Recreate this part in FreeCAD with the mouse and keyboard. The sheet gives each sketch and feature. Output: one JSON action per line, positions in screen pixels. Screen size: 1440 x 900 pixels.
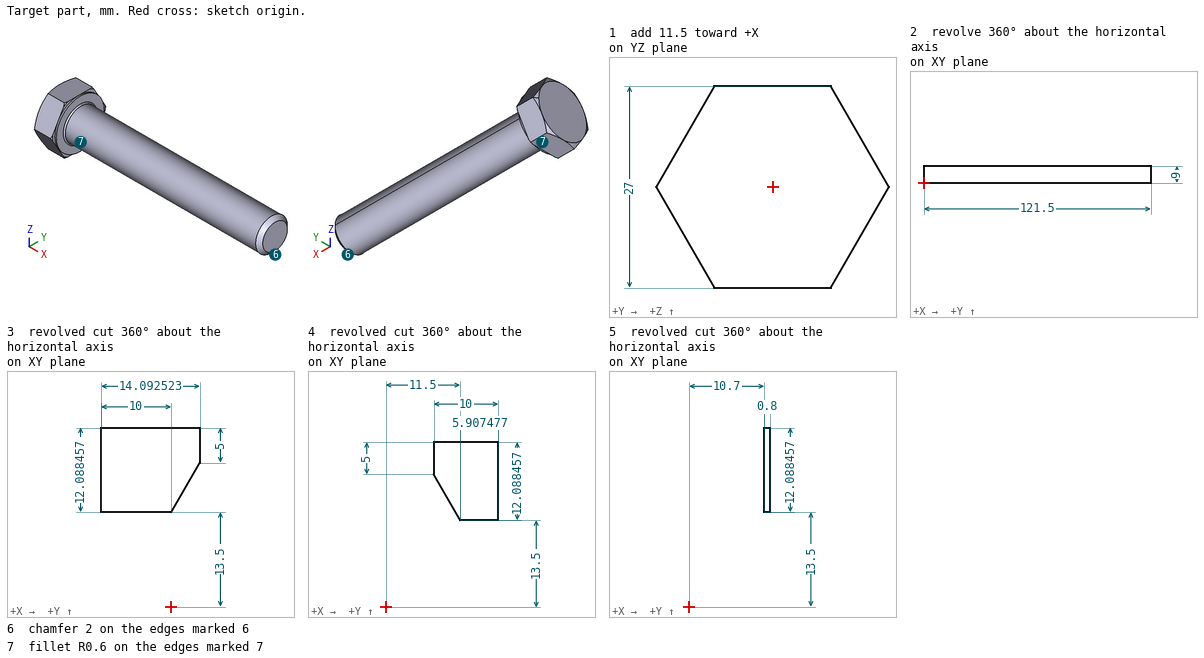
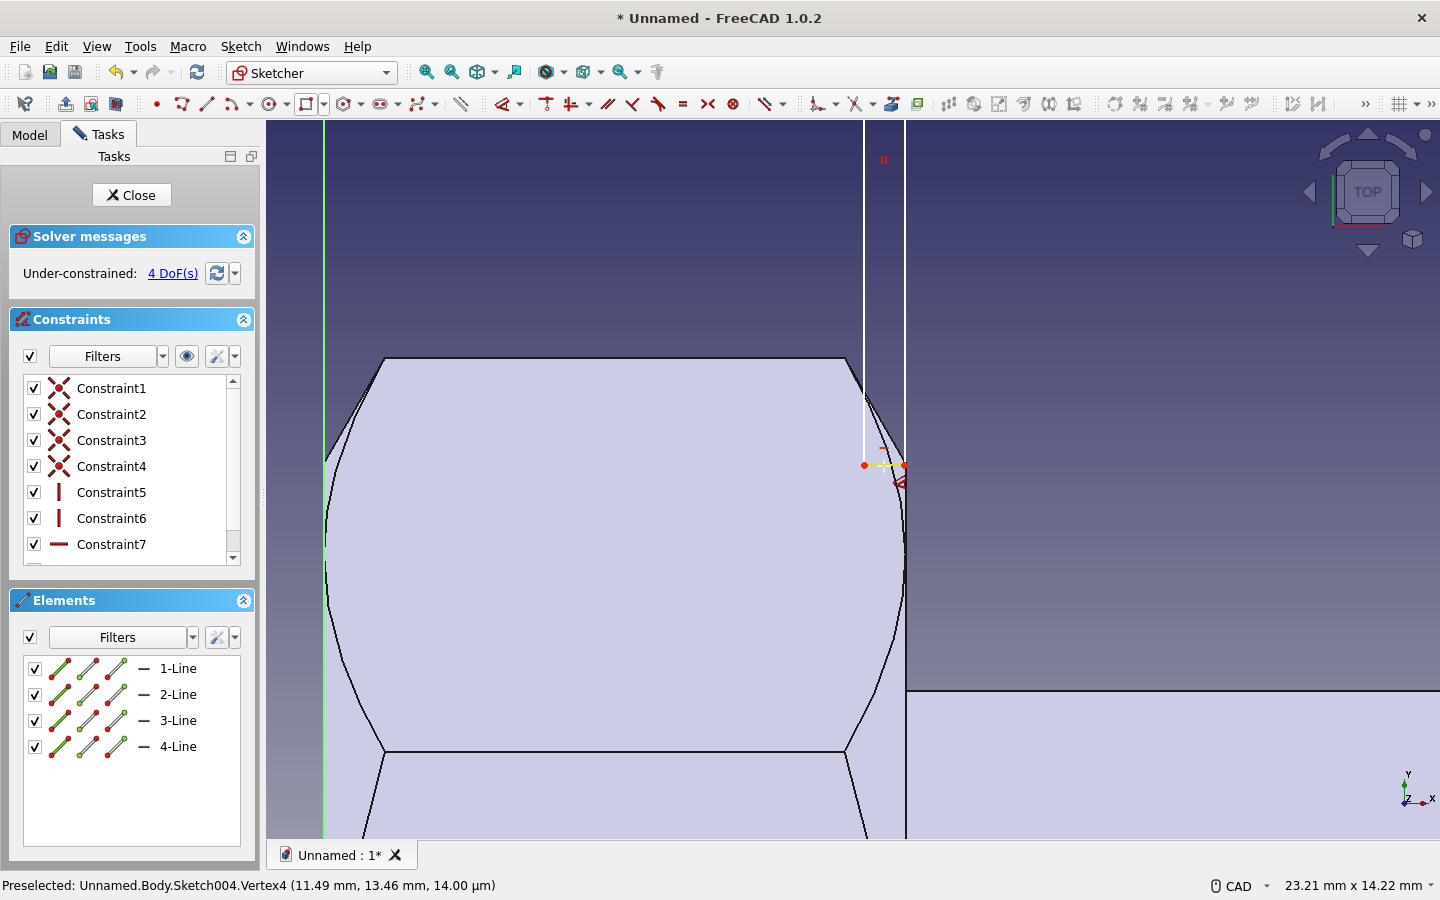
{"action": "left_click", "coordinate": [884, 465]}
{"action": "left_click", "coordinate": [884, 431]}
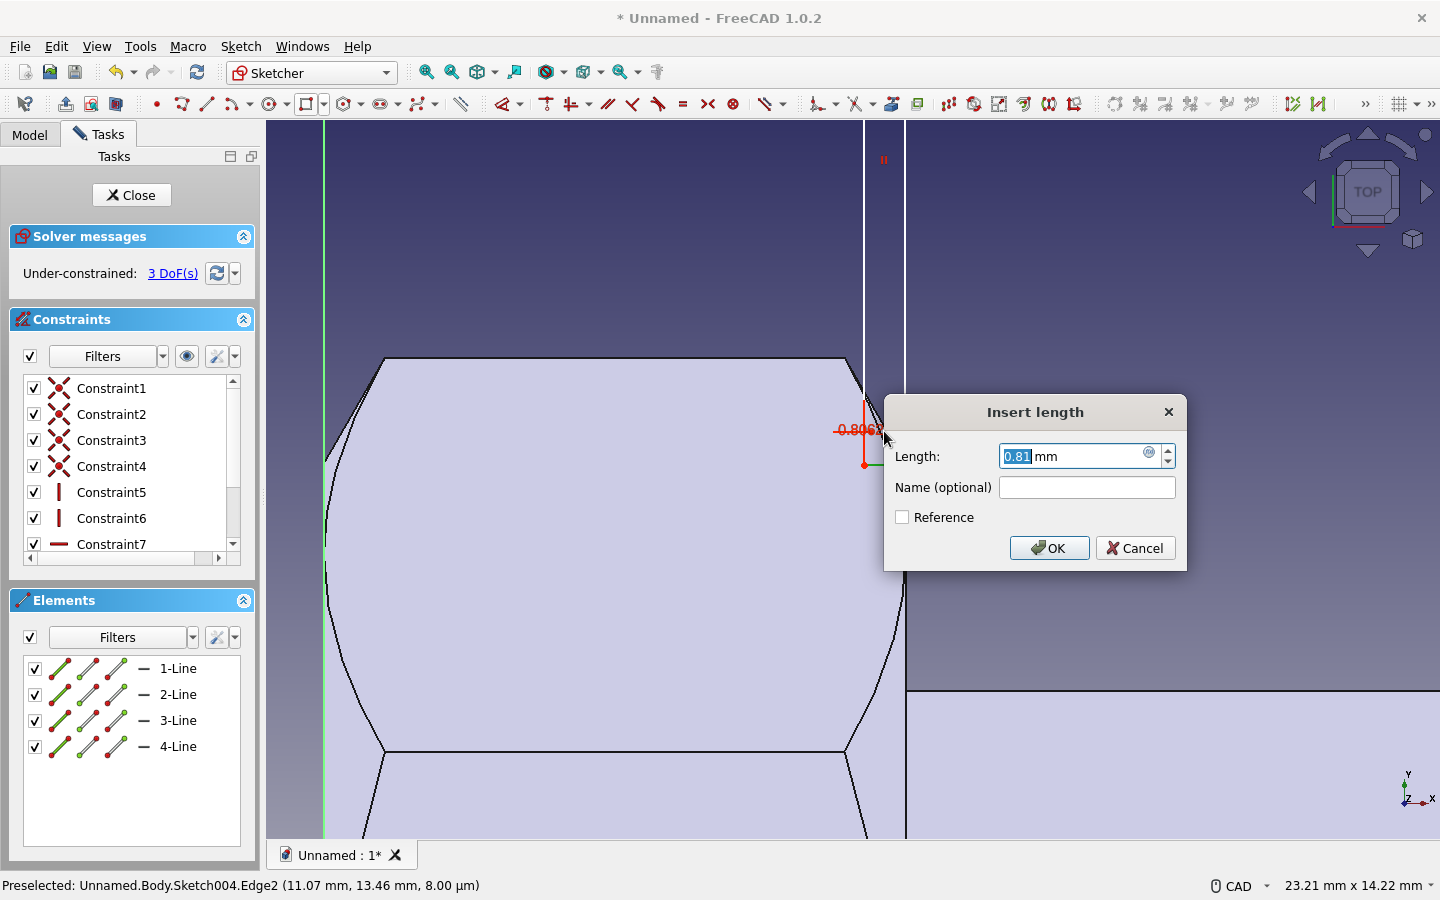
{"action": "type", "text": "0.8"}
{"action": "key", "text": "Return"}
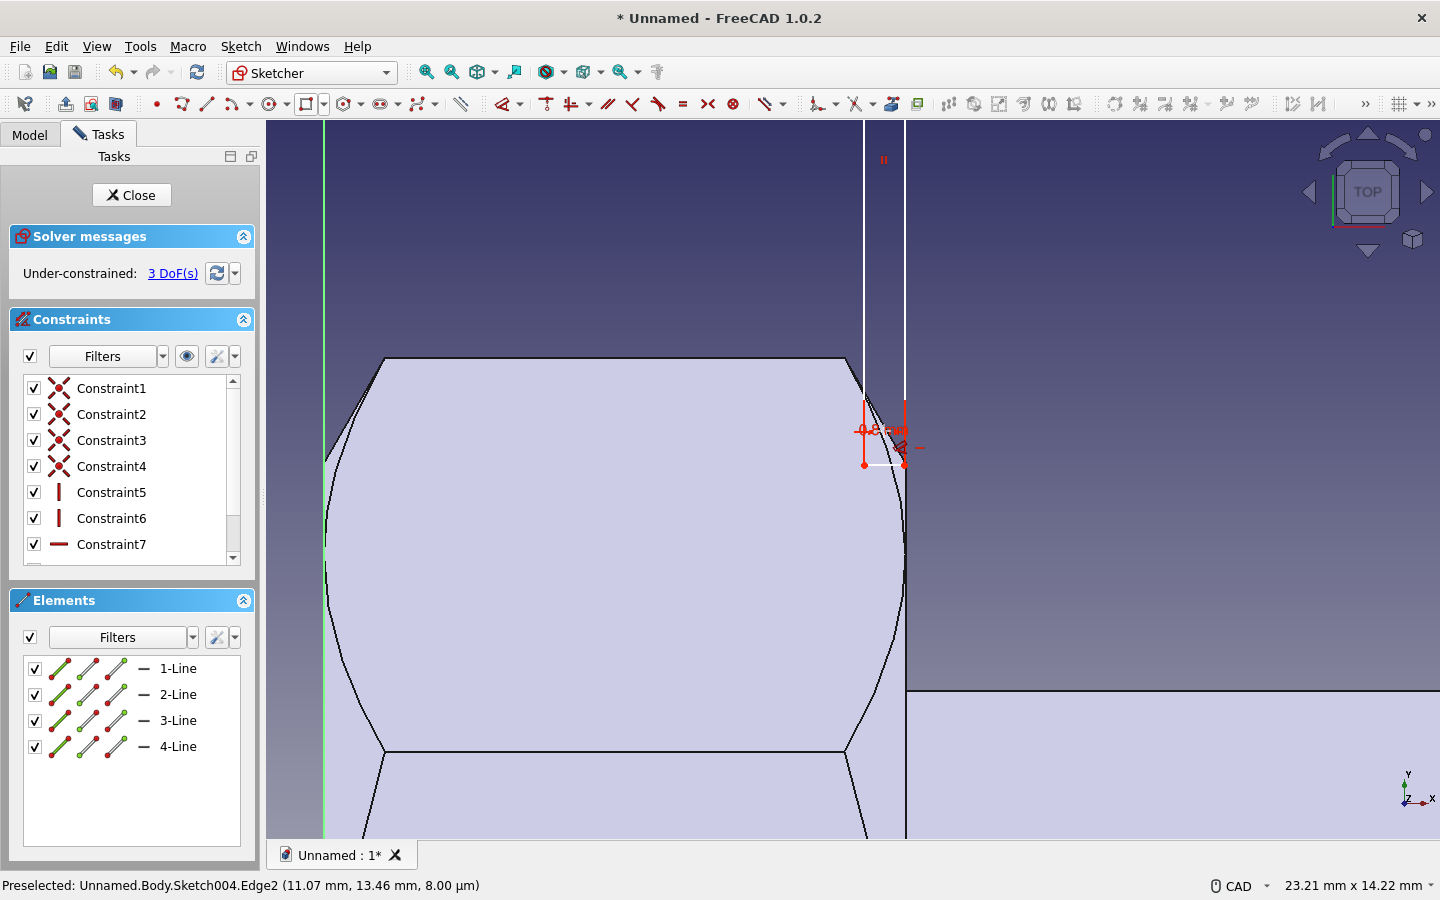
{"action": "scroll", "coordinate": [883, 468], "scroll_direction": "down", "scroll_amount": 5}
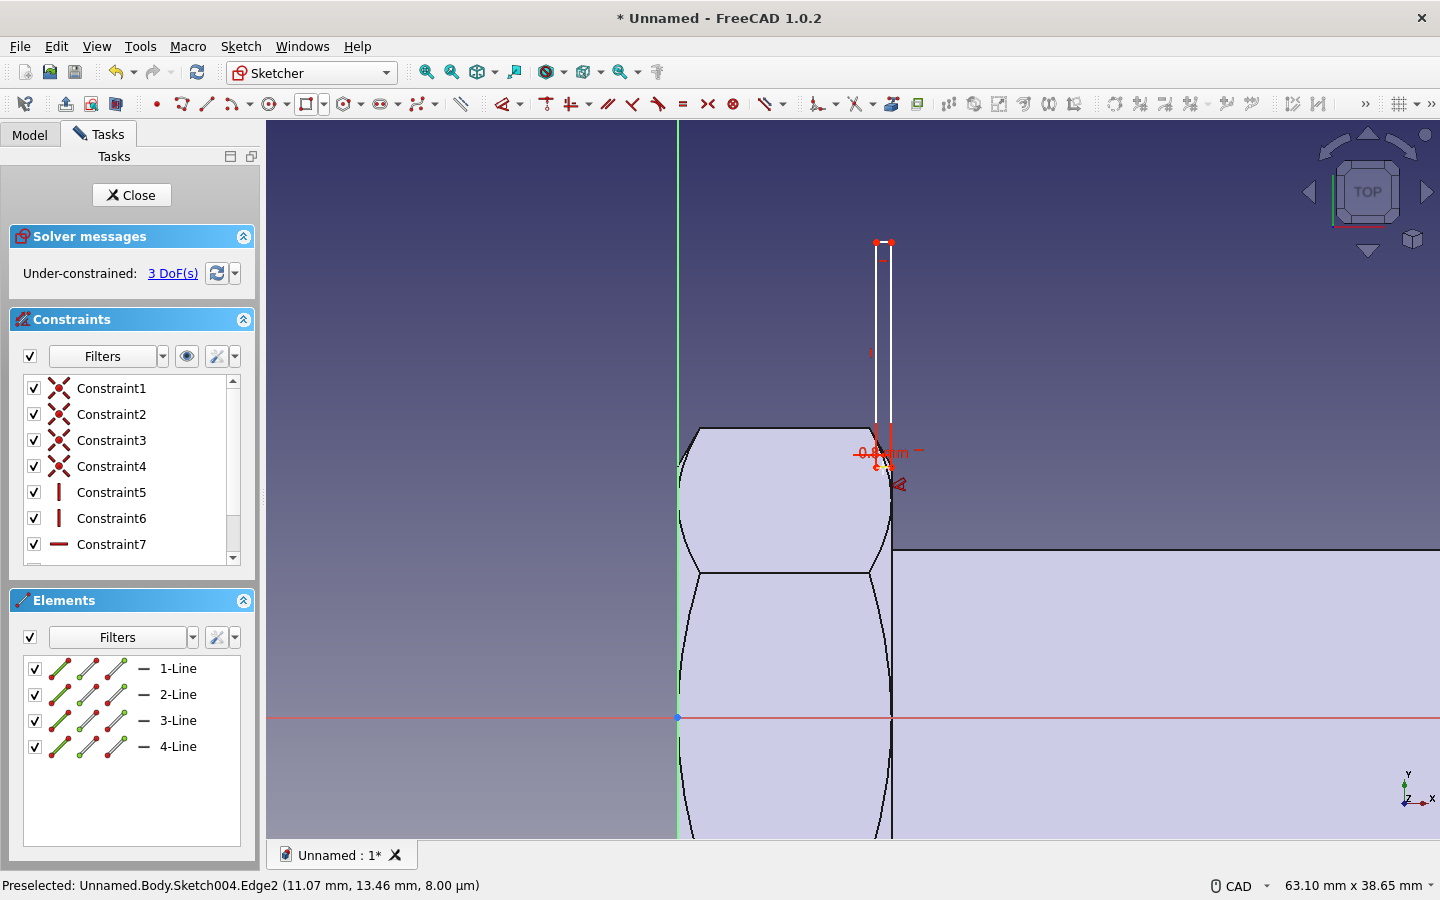
{"action": "left_click", "coordinate": [876, 242]}
{"action": "left_click", "coordinate": [777, 752]}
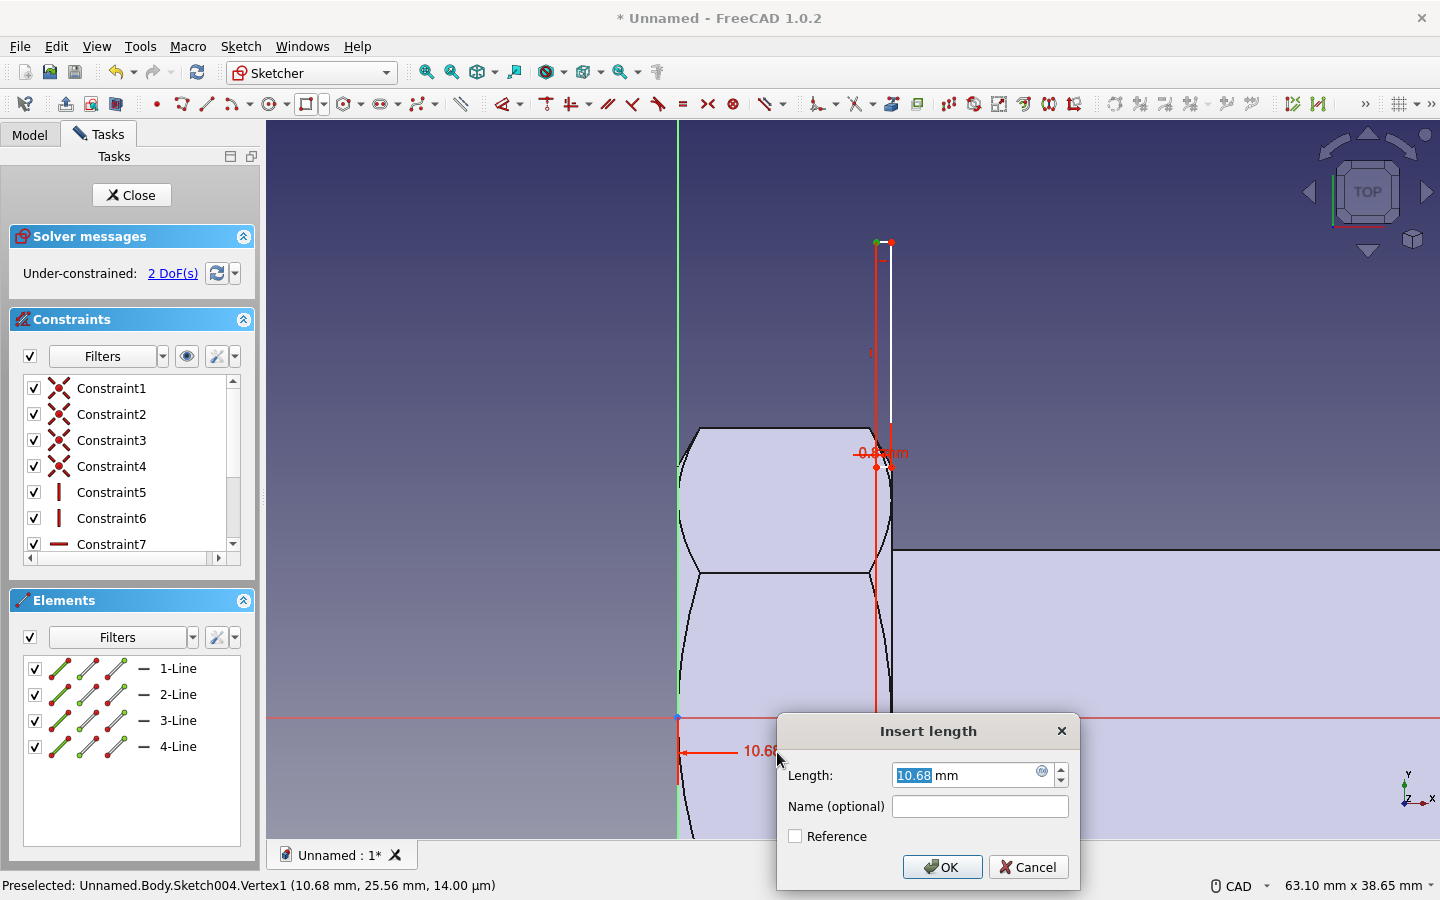
{"action": "type", "text": "10.7"}
{"action": "key", "text": "Return"}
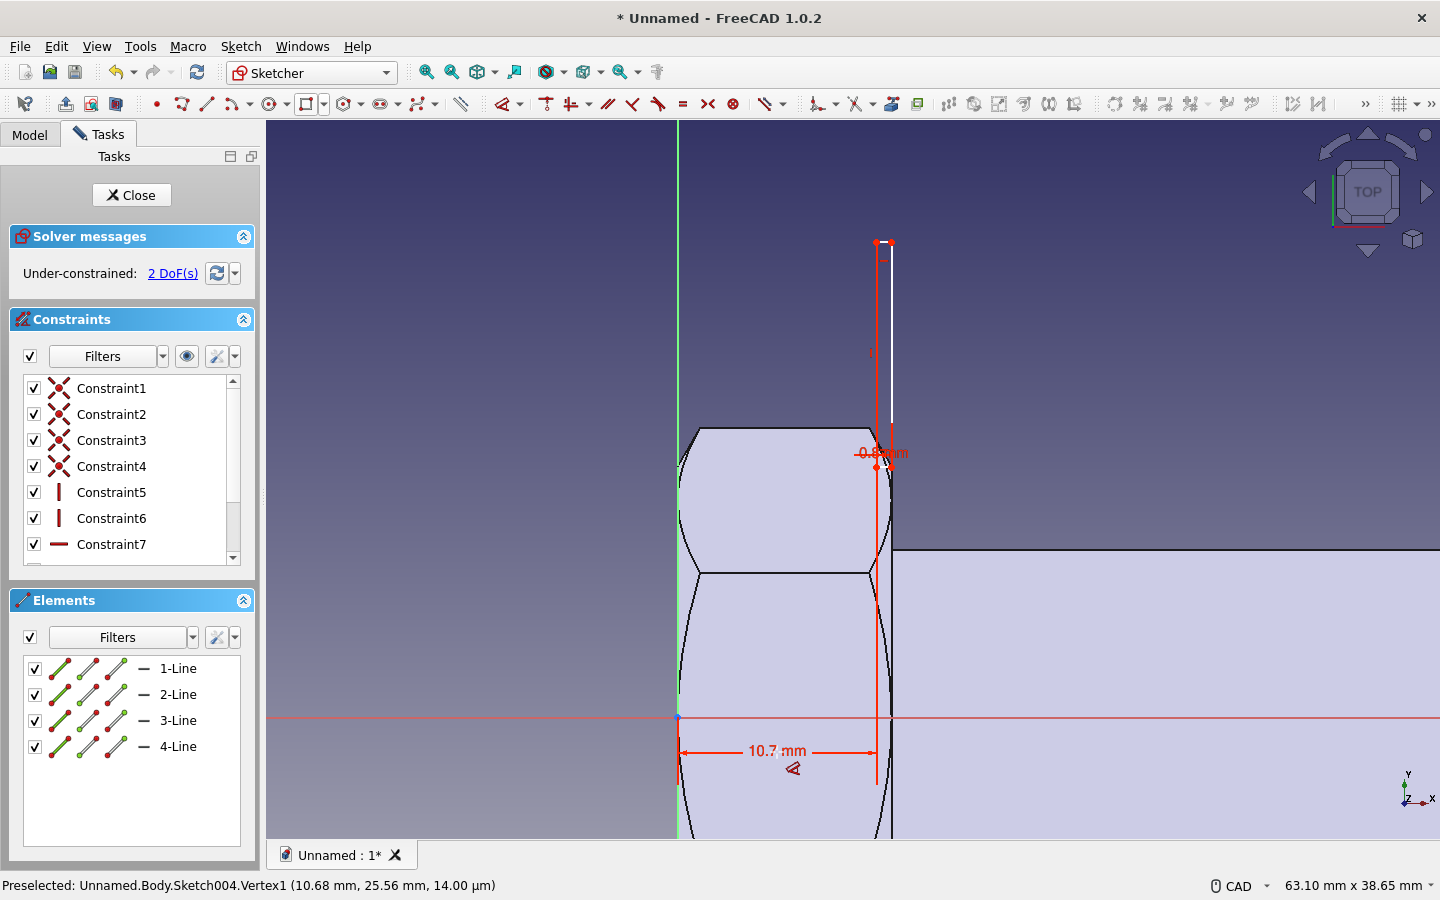
{"action": "left_click", "coordinate": [877, 467]}
{"action": "left_click", "coordinate": [644, 593]}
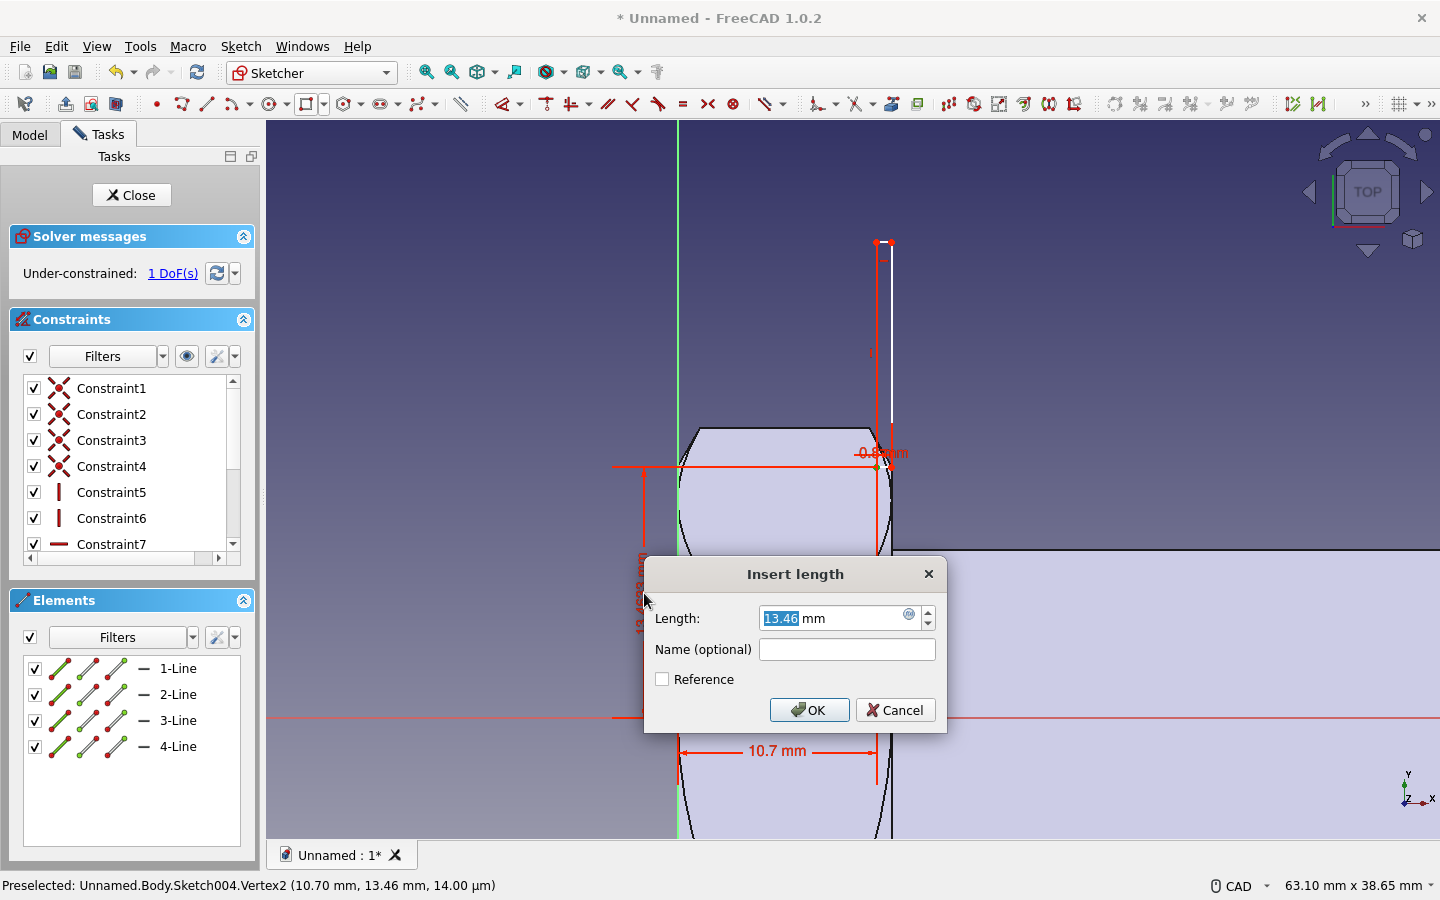
{"action": "type", "text": "13.5"}
{"action": "key", "text": "Return"}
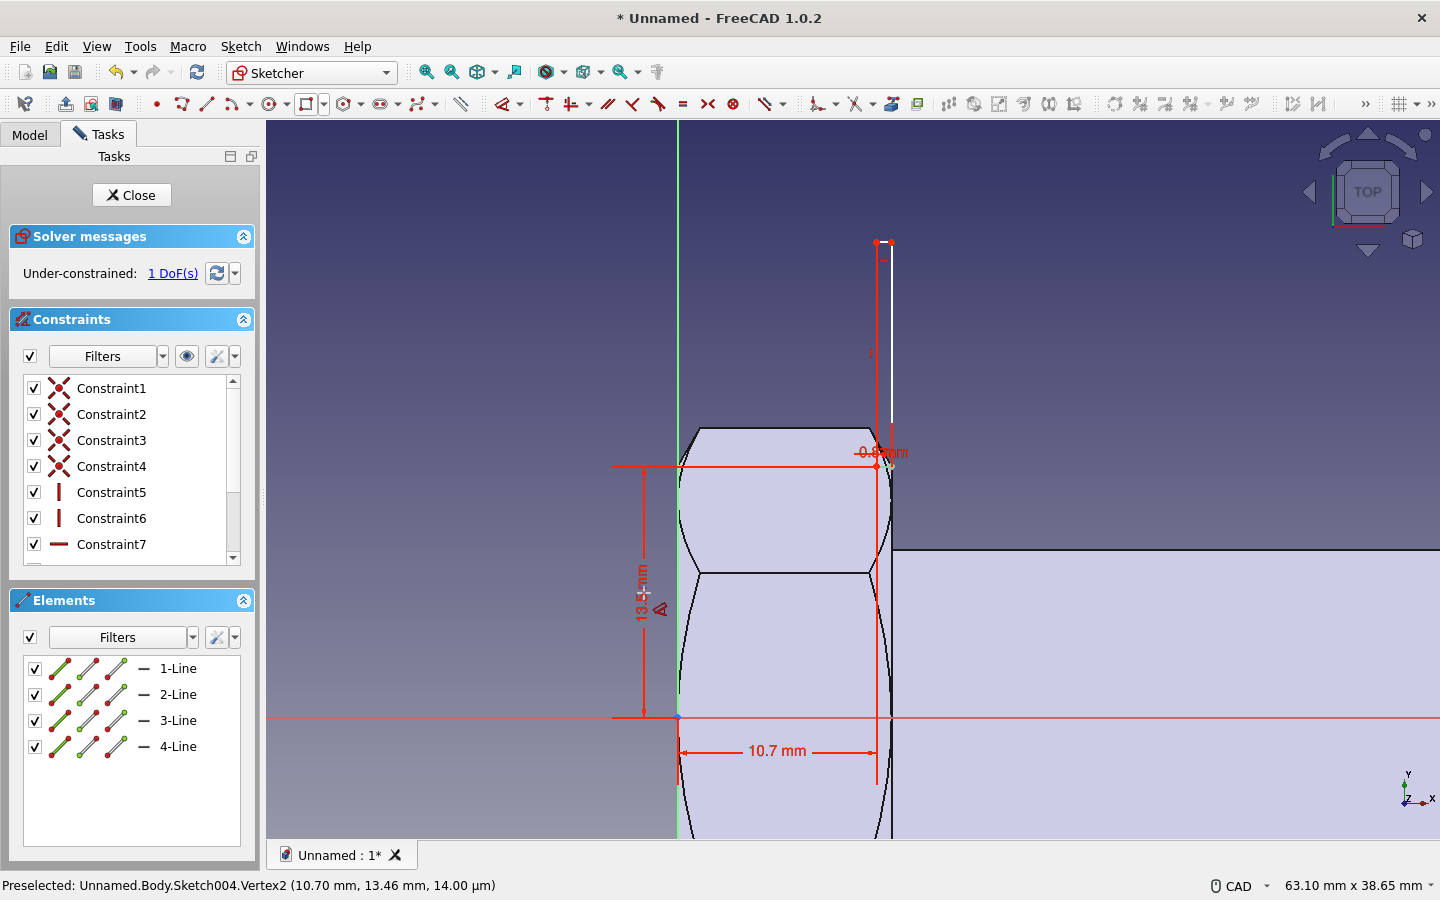
{"action": "left_click", "coordinate": [877, 310]}
{"action": "left_click", "coordinate": [911, 354]}